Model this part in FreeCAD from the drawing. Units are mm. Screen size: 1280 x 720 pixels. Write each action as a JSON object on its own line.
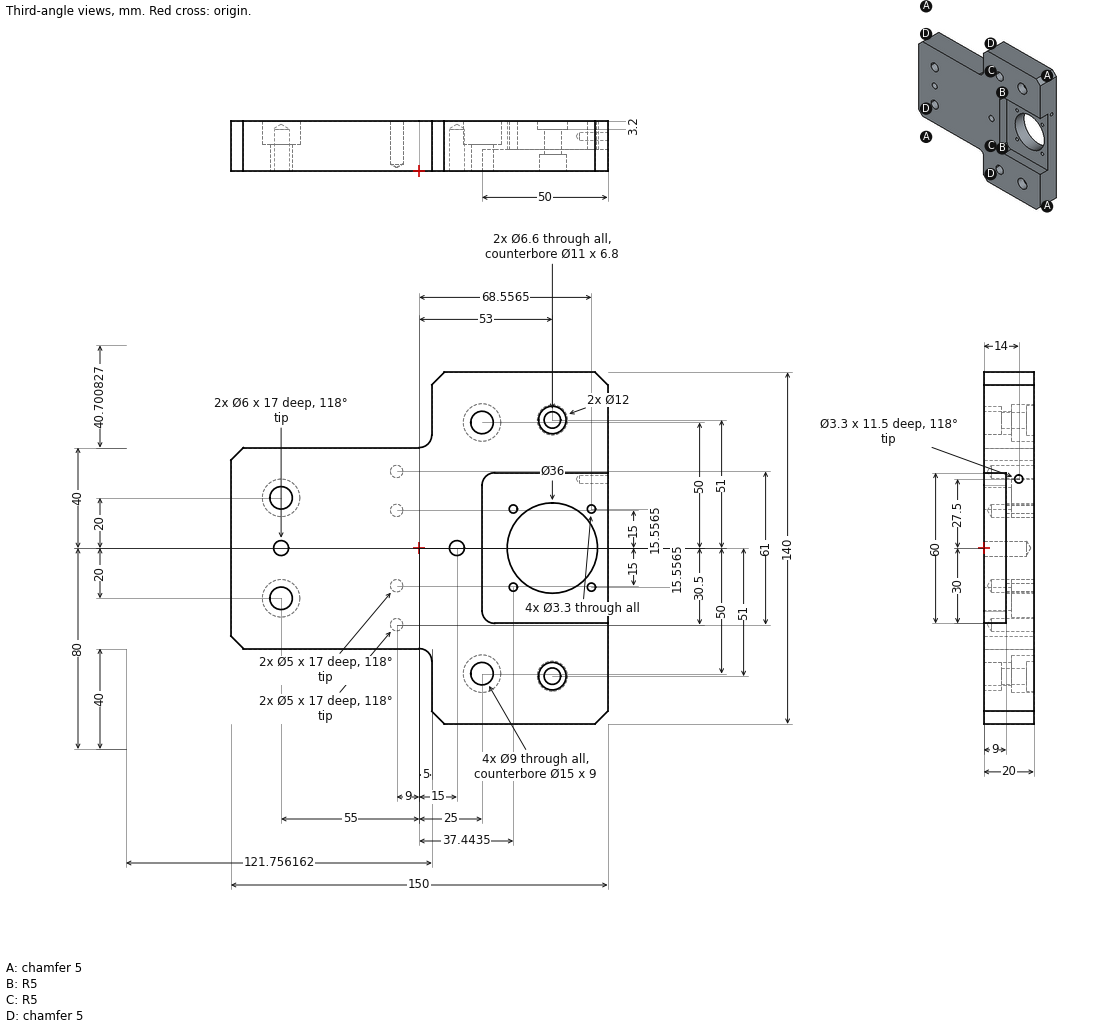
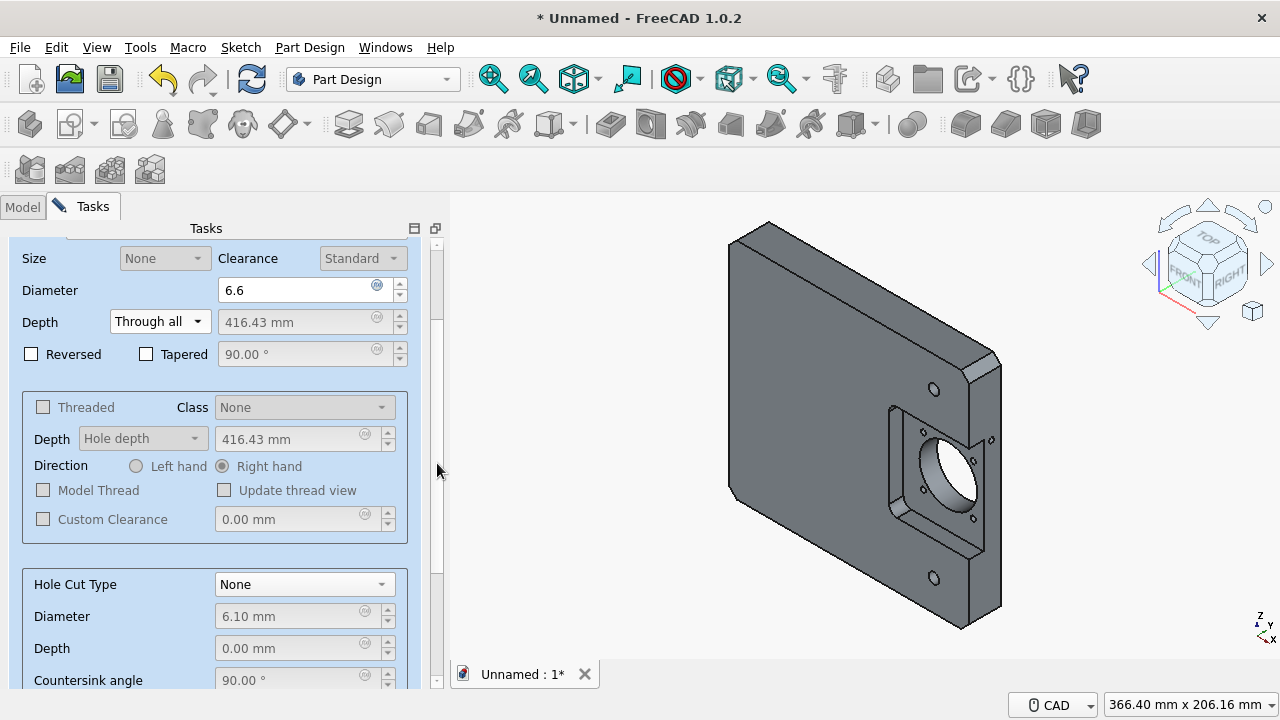
{"action": "left_click", "coordinate": [306, 584]}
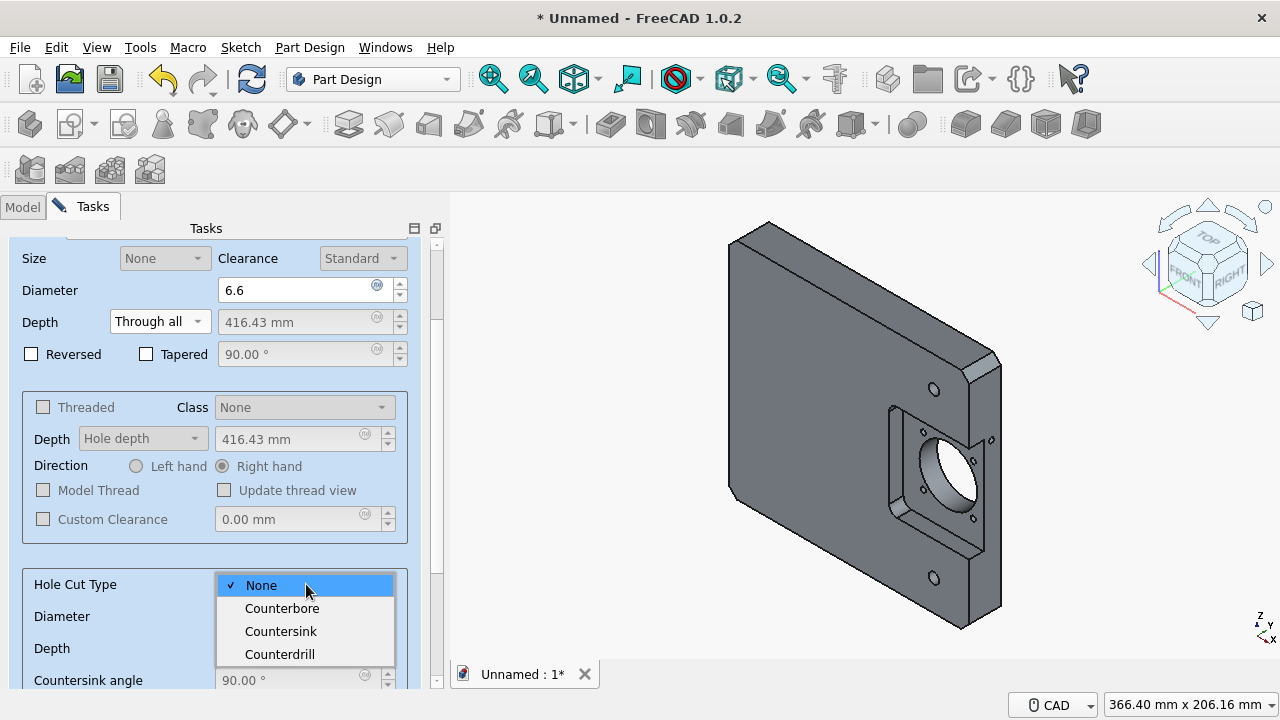
{"action": "left_click", "coordinate": [304, 608]}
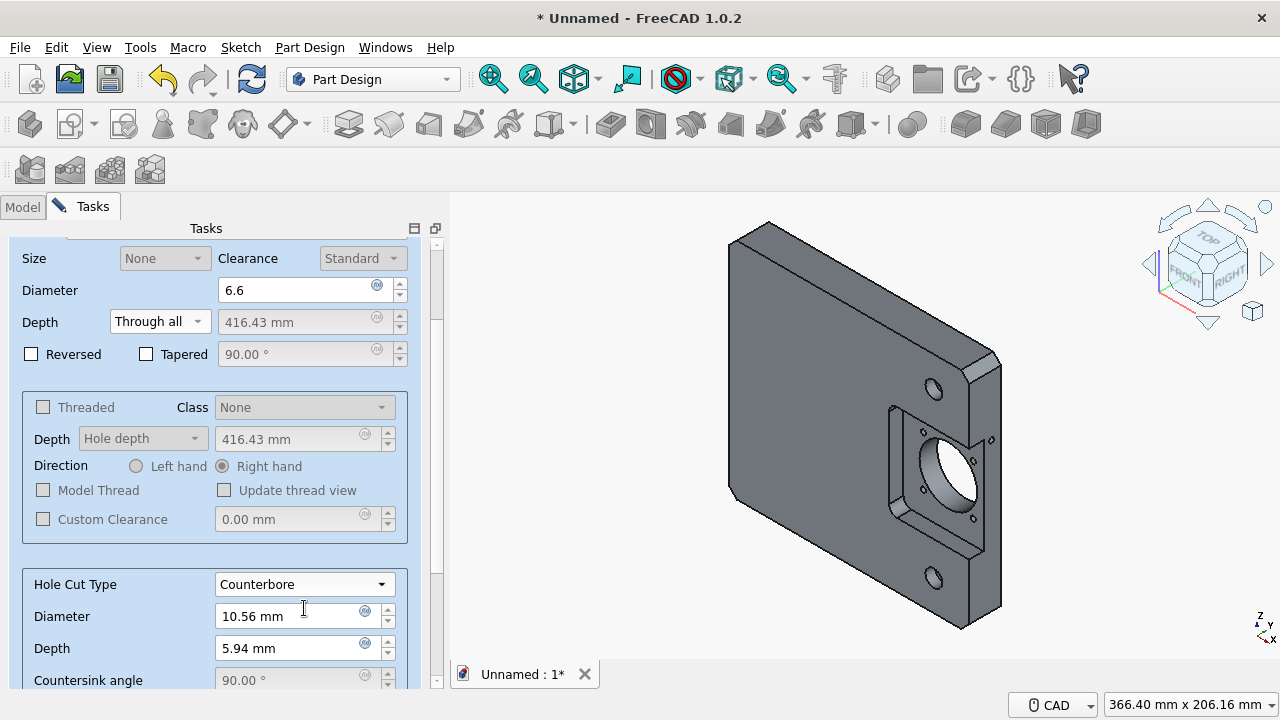
{"action": "triple_click", "coordinate": [298, 616]}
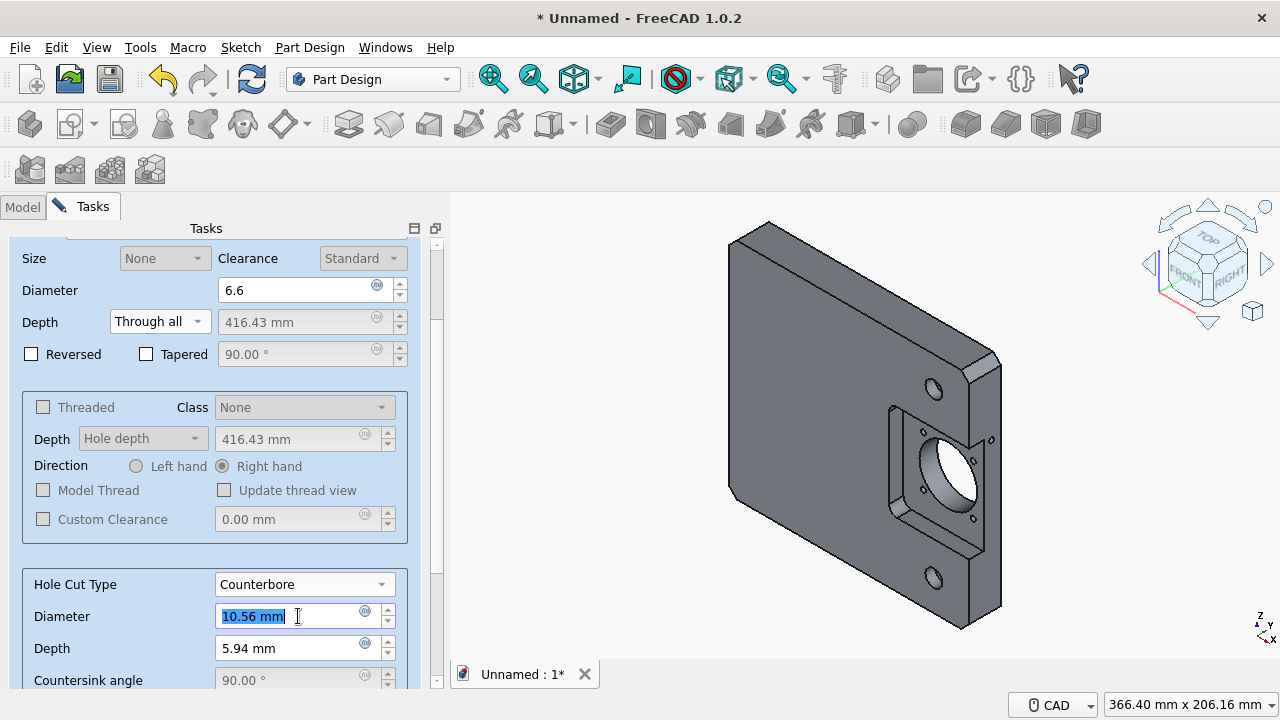
{"action": "type", "text": "11"}
{"action": "key", "text": "Tab"}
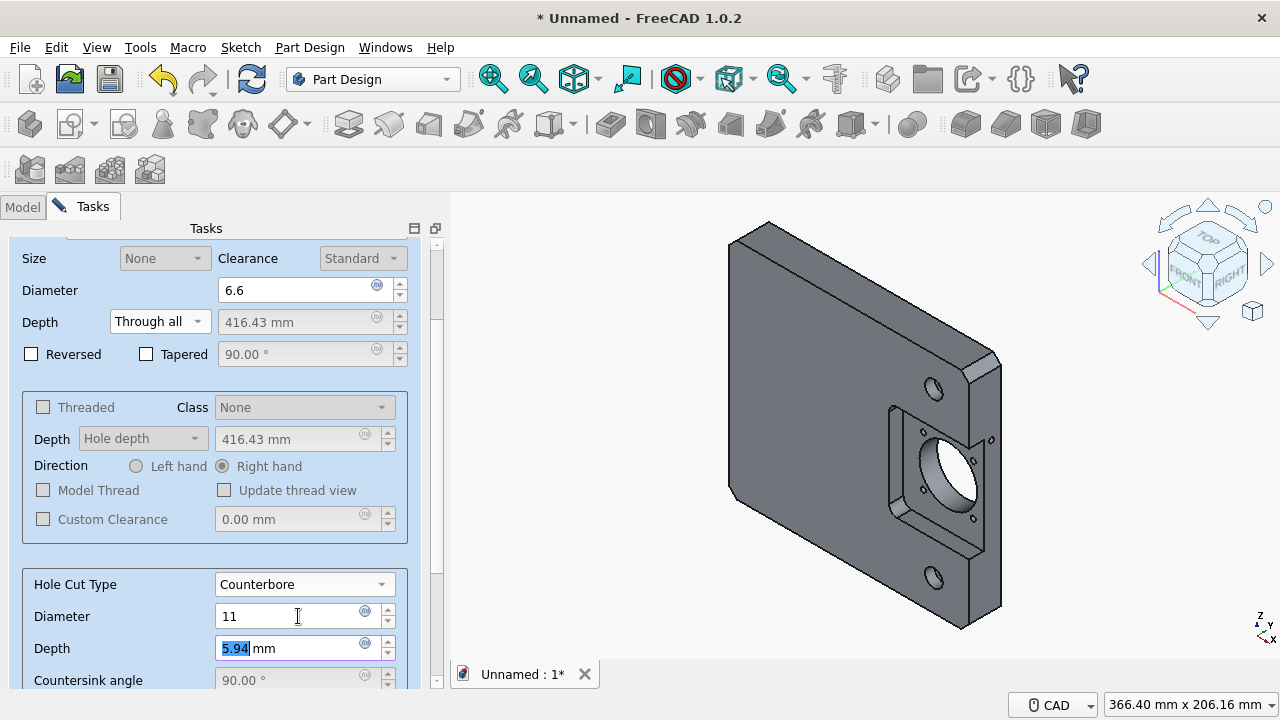
{"action": "type", "text": "6.8"}
{"action": "key", "text": "Tab"}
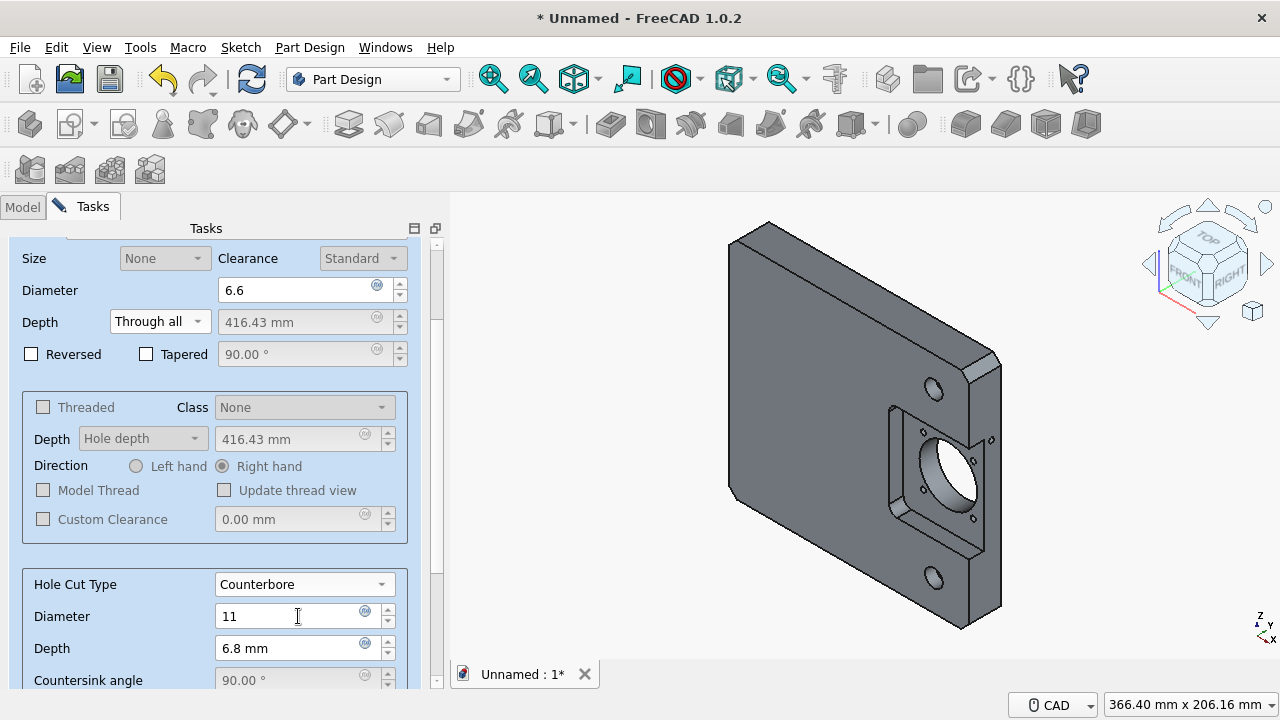
{"action": "scroll", "coordinate": [437, 463], "scroll_direction": "up", "scroll_amount": 3}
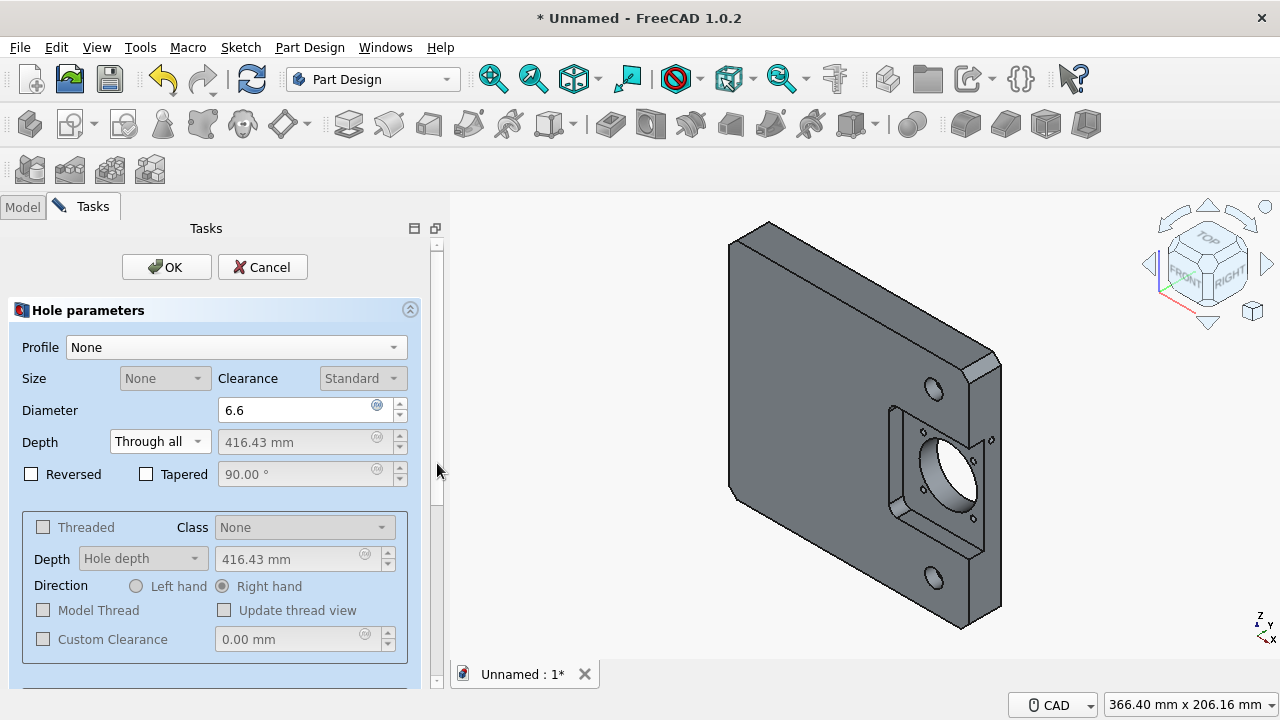
{"action": "left_click", "coordinate": [167, 267]}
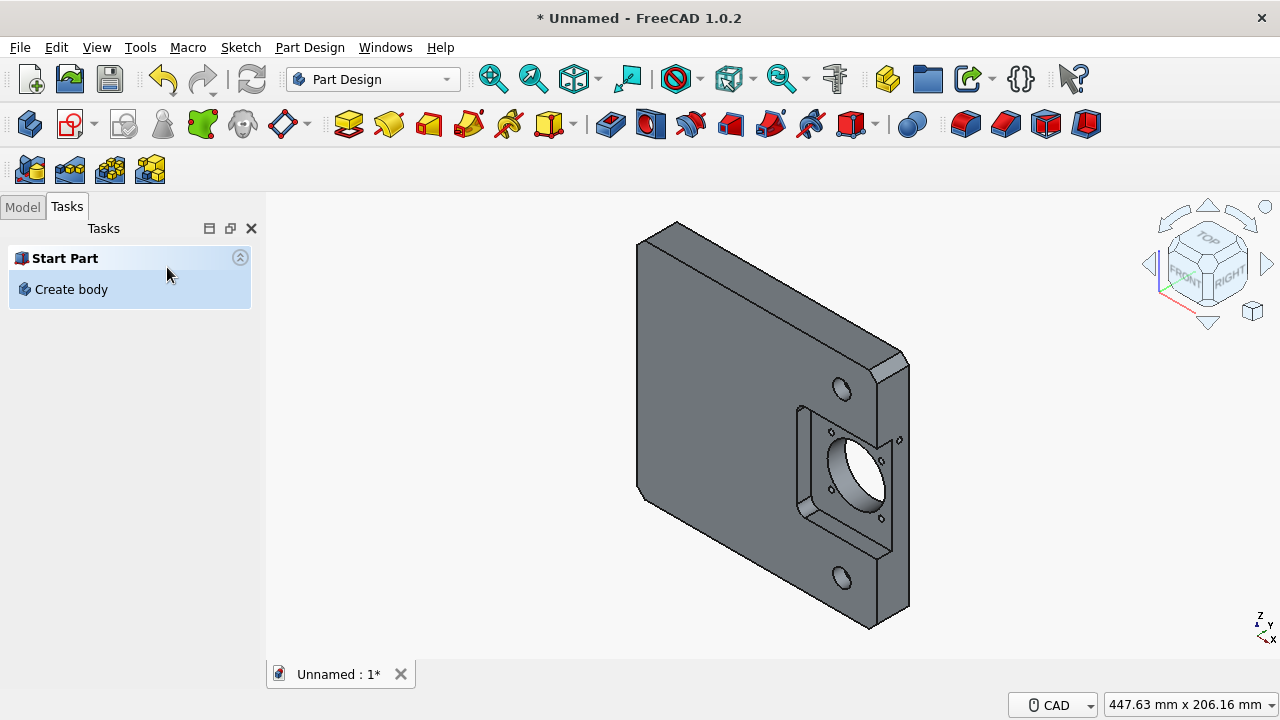
{"action": "key", "text": "4"}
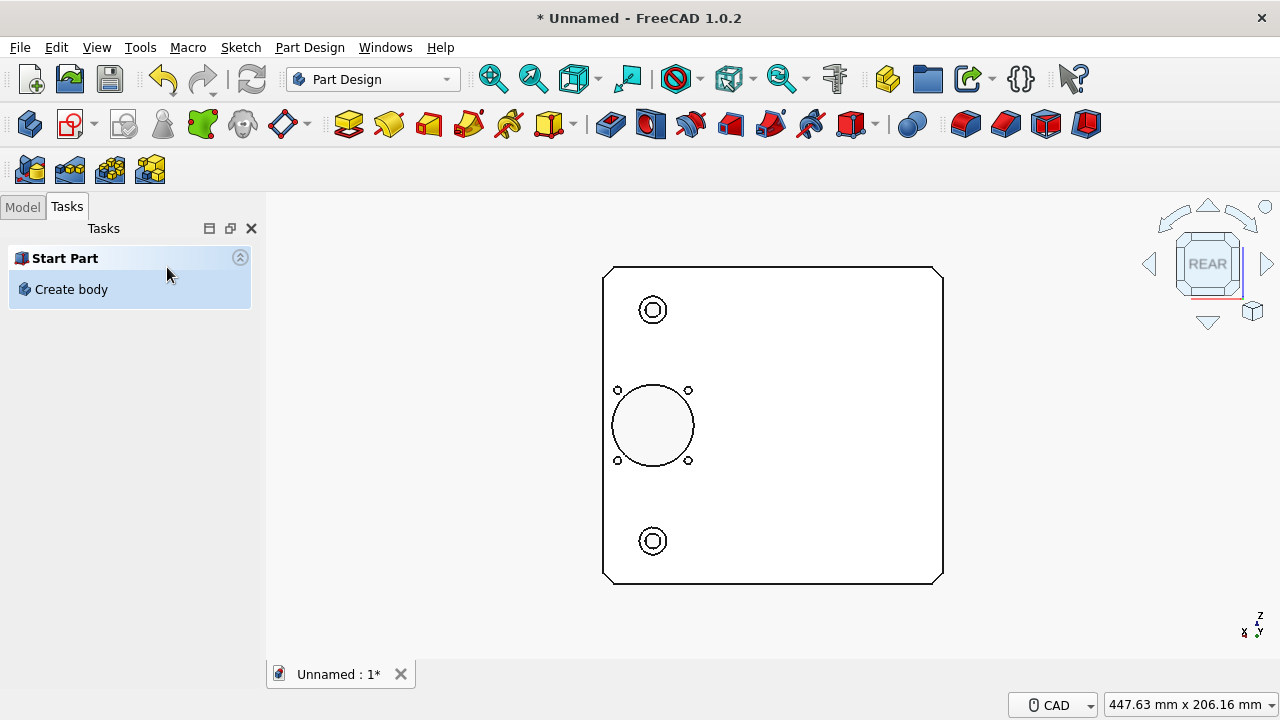
{"action": "left_click", "coordinate": [822, 425]}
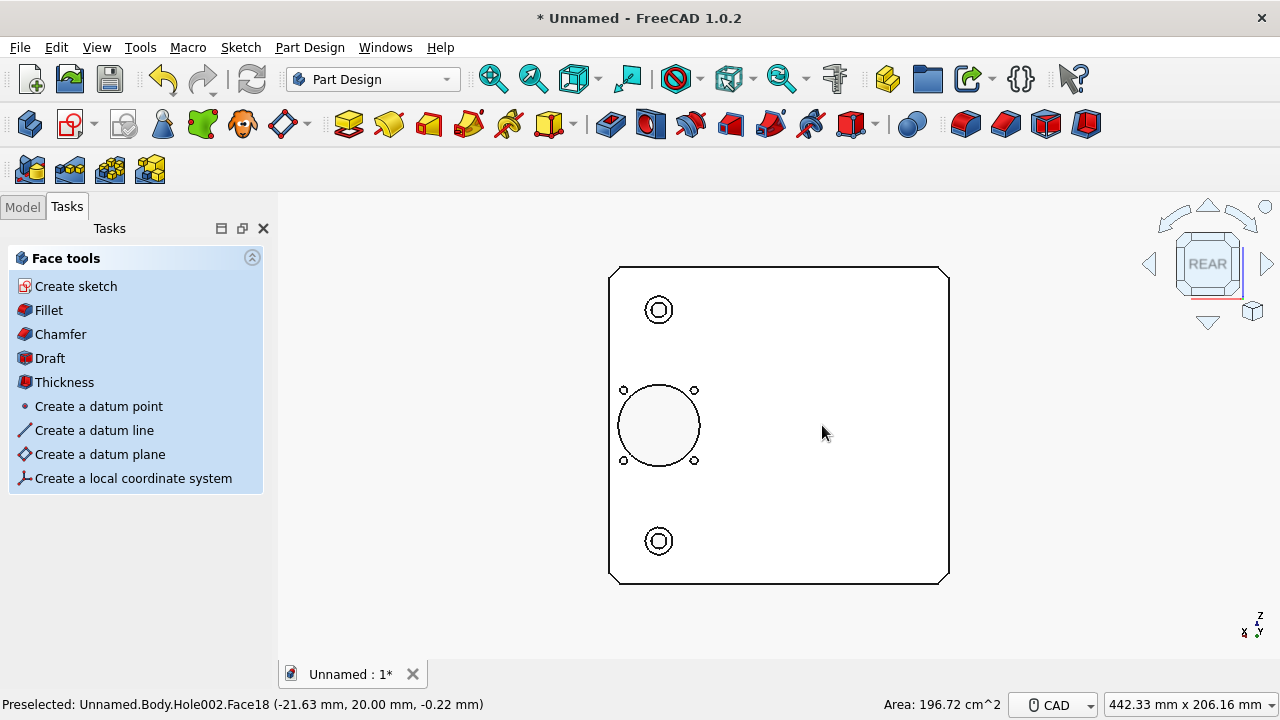
{"action": "left_click", "coordinate": [70, 124]}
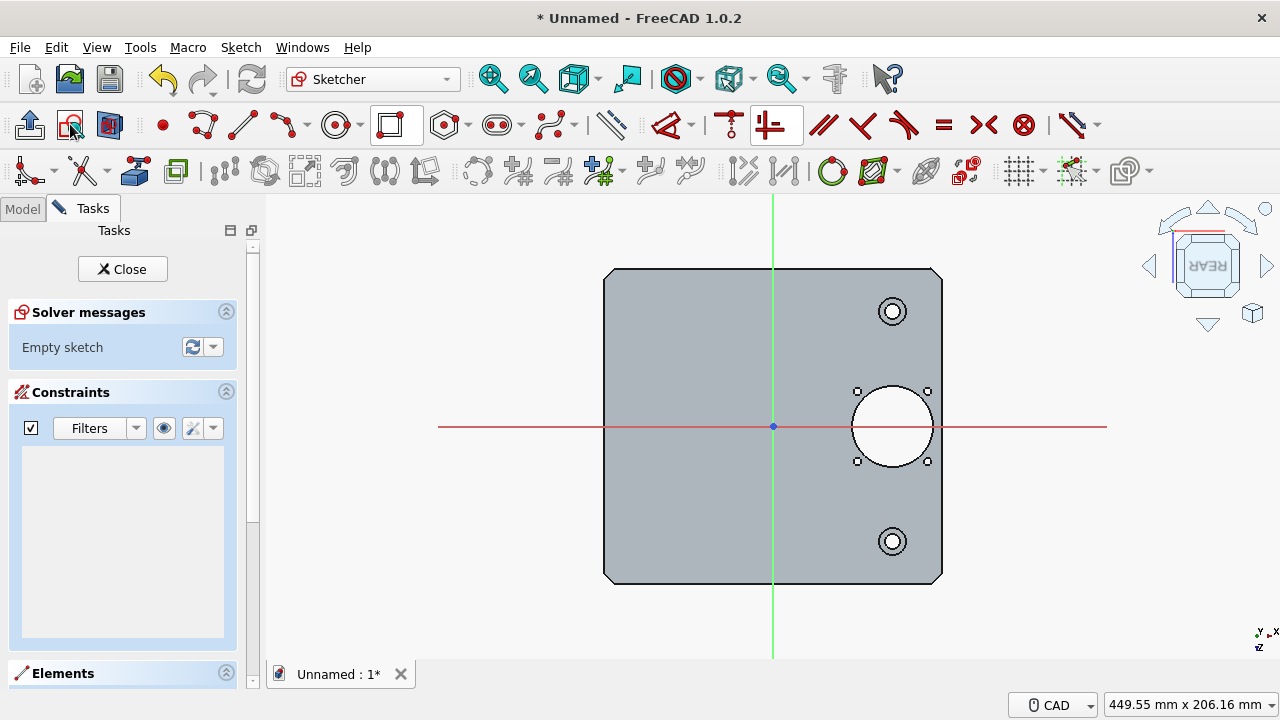
{"action": "scroll", "coordinate": [964, 423], "scroll_direction": "down", "scroll_amount": 1}